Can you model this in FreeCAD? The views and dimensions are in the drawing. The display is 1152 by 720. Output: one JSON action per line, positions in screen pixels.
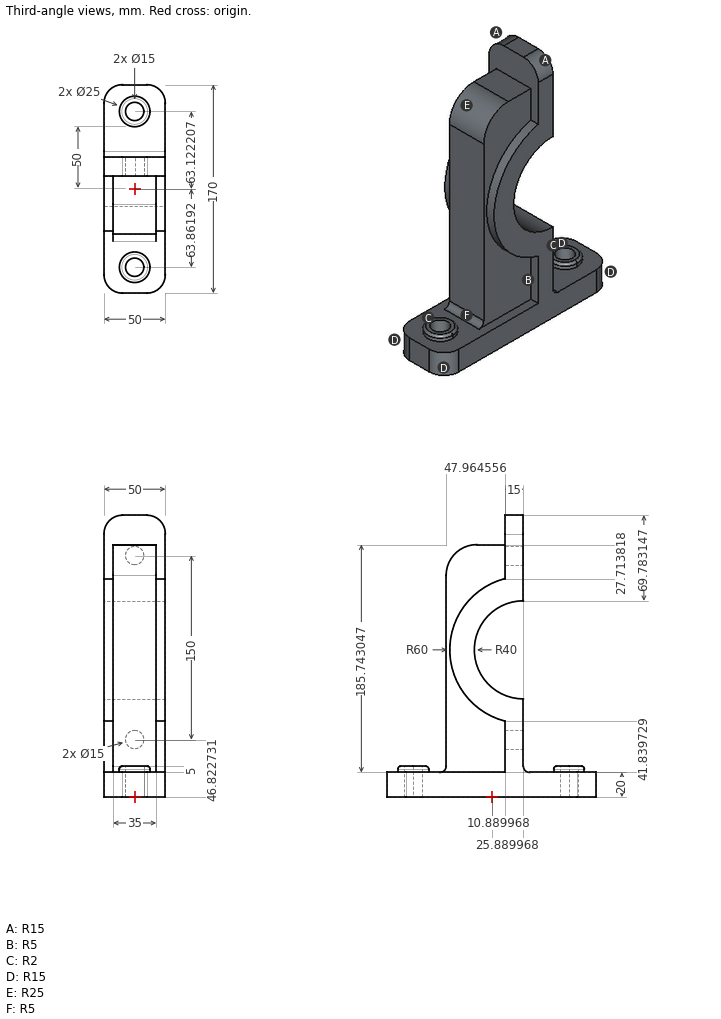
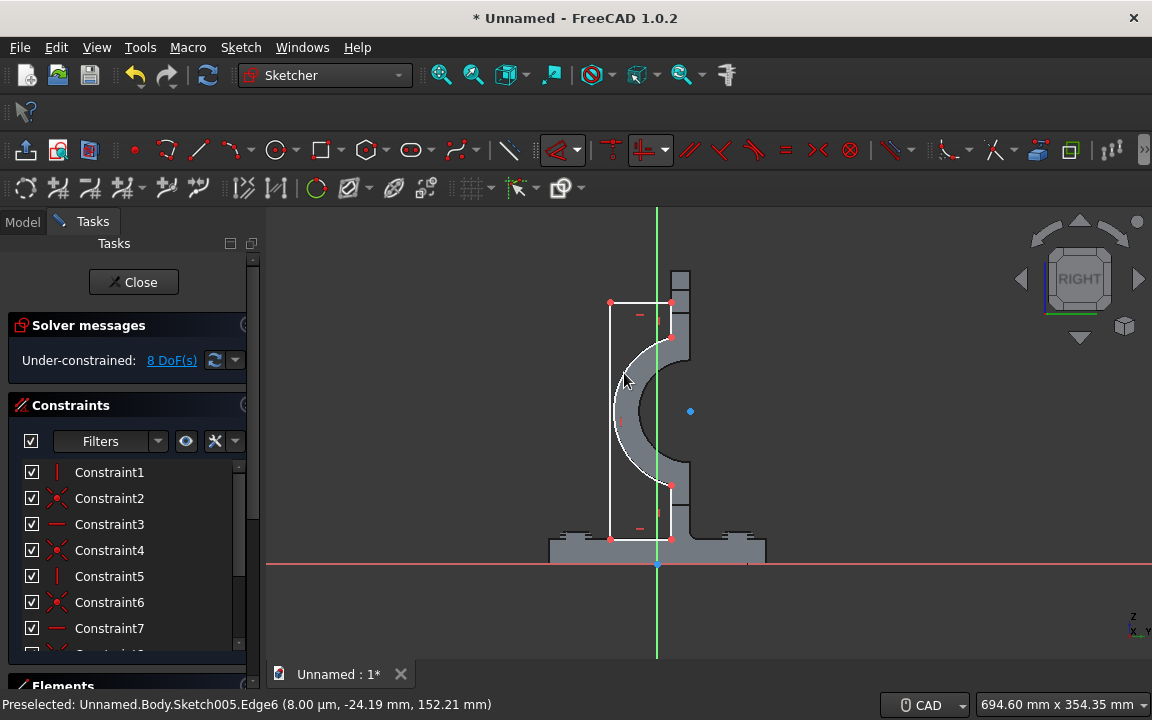
{"action": "left_click", "coordinate": [624, 374]}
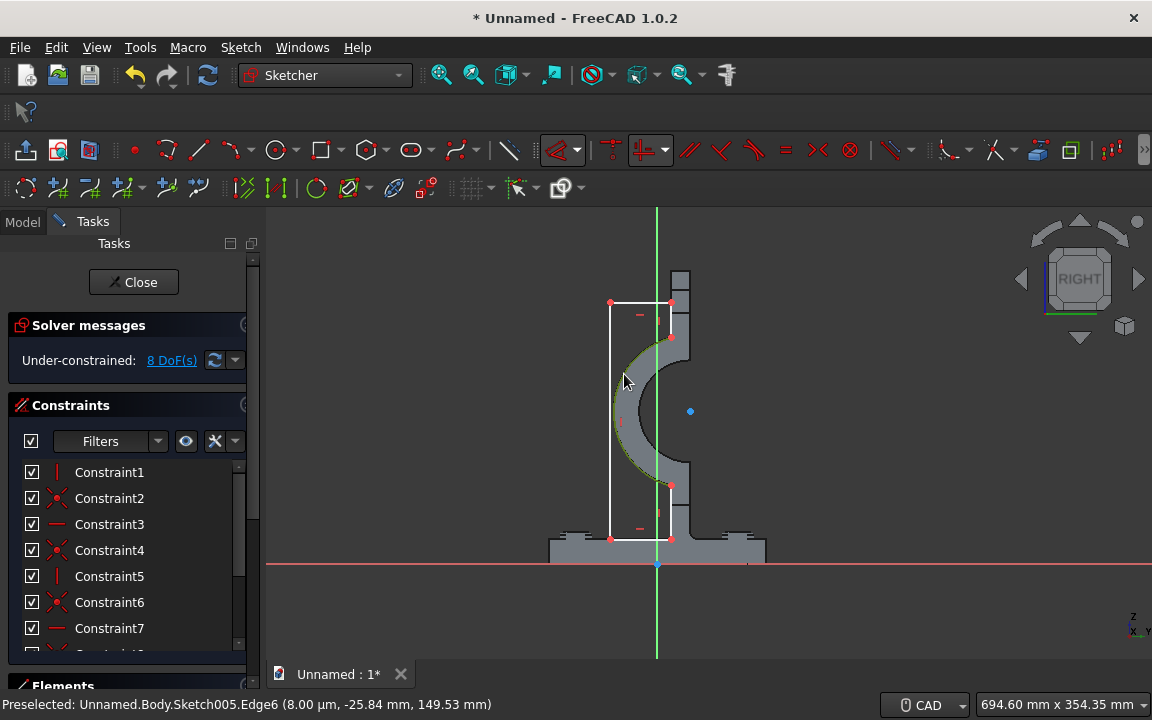
{"action": "key", "text": "k r"}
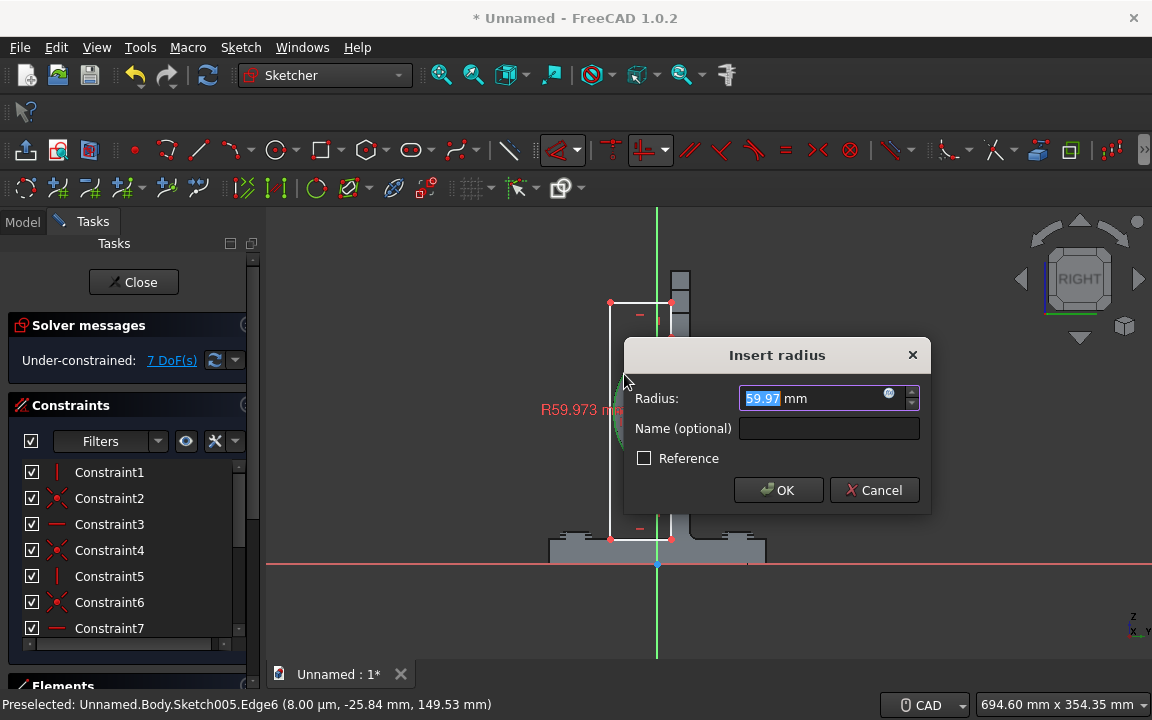
{"action": "type", "text": "60"}
{"action": "key", "text": "Return"}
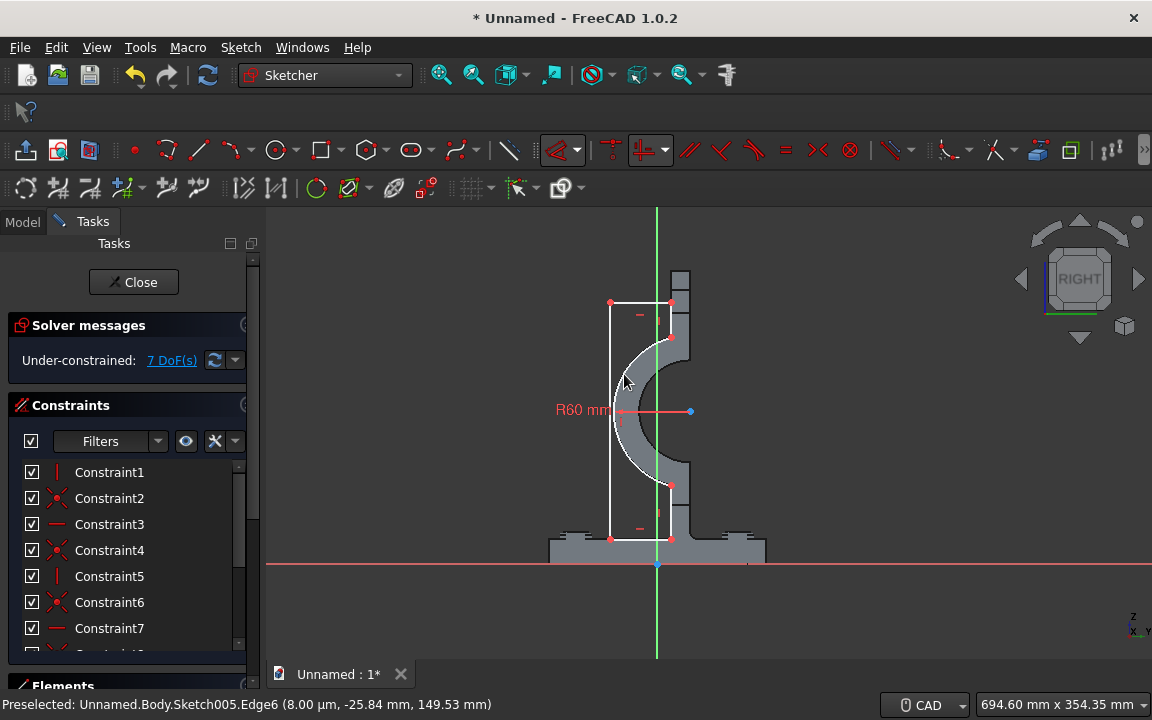
{"action": "scroll", "coordinate": [610, 540], "scroll_direction": "up", "scroll_amount": 3}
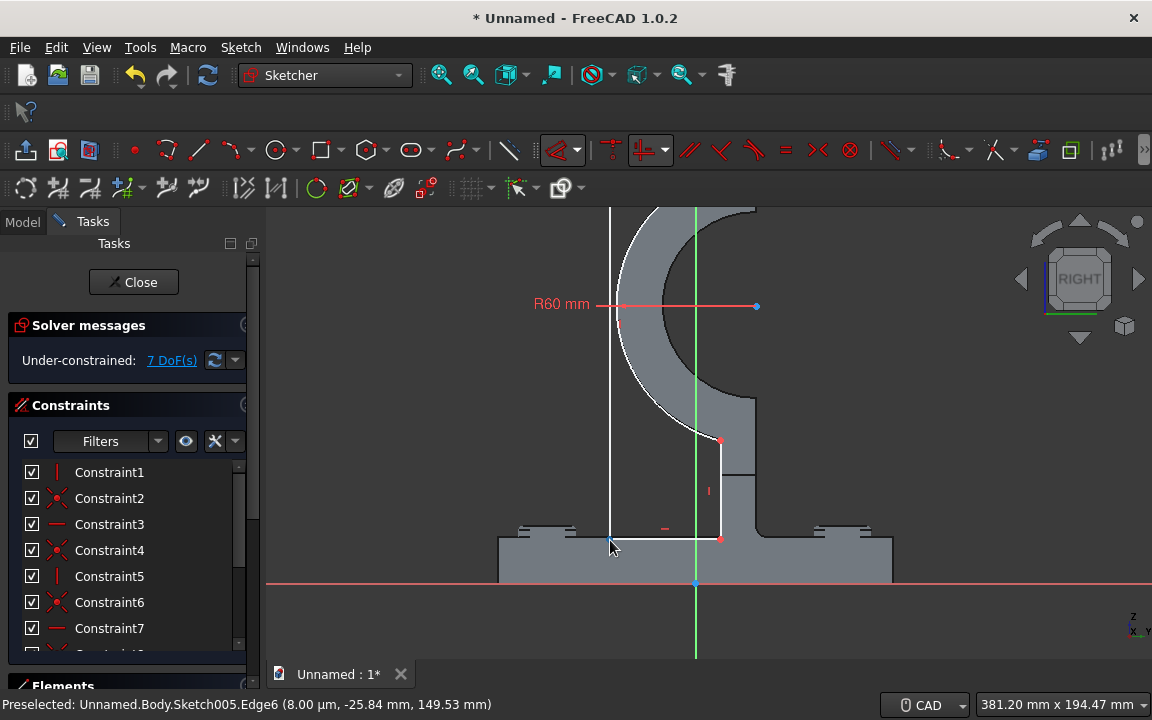
{"action": "left_click", "coordinate": [610, 539]}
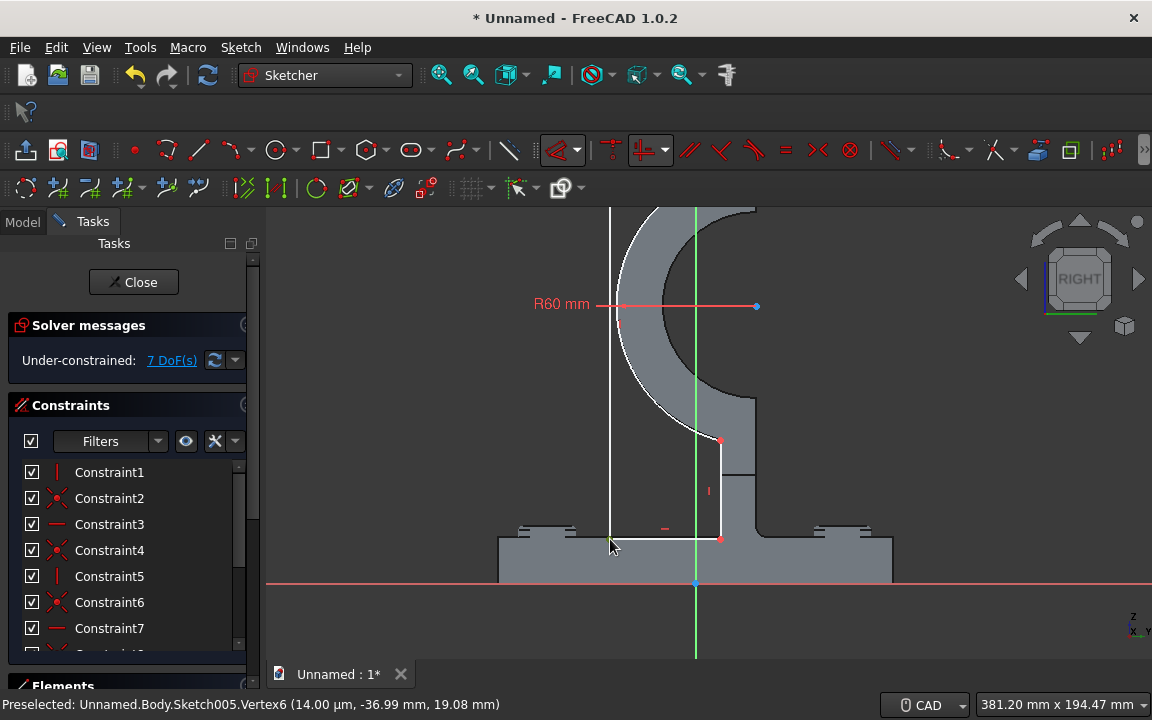
{"action": "left_click", "coordinate": [580, 150]}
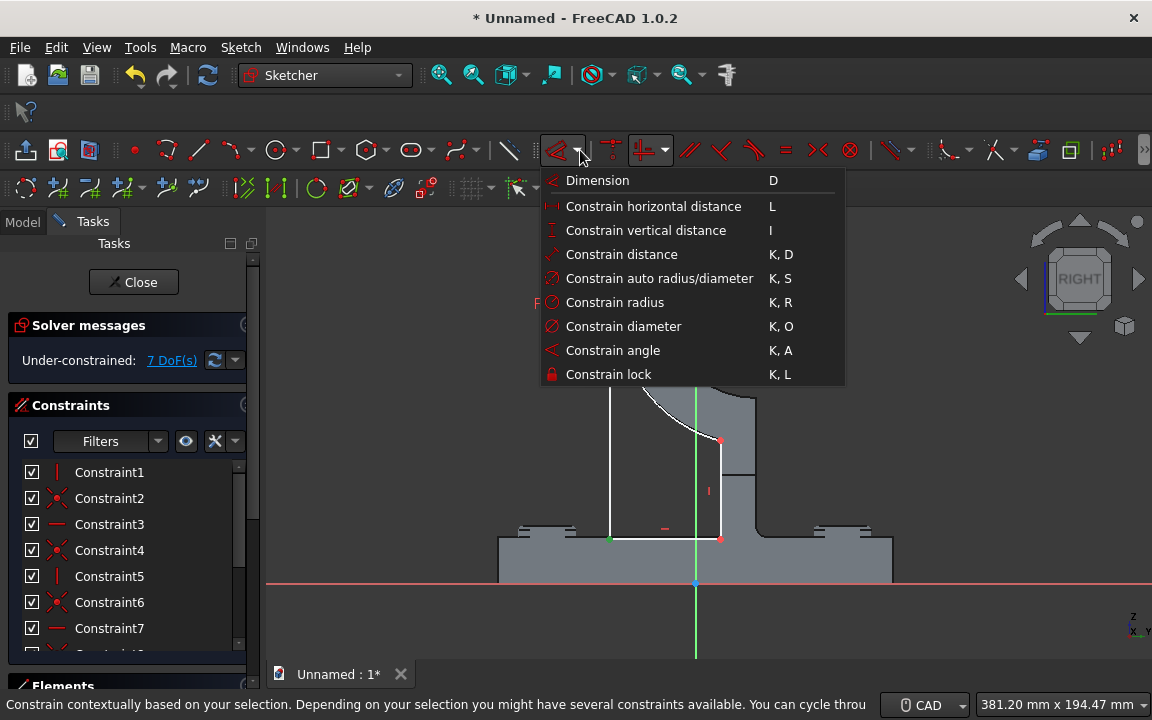
{"action": "left_click", "coordinate": [693, 230]}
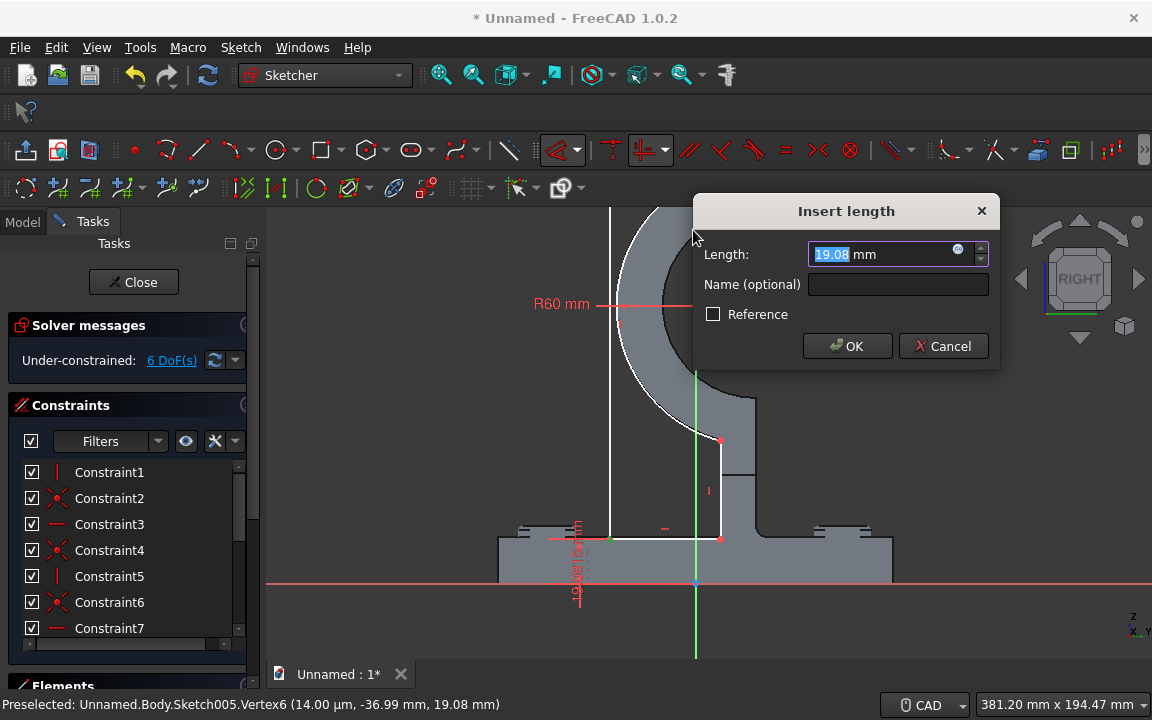
{"action": "type", "text": "20"}
{"action": "key", "text": "Return"}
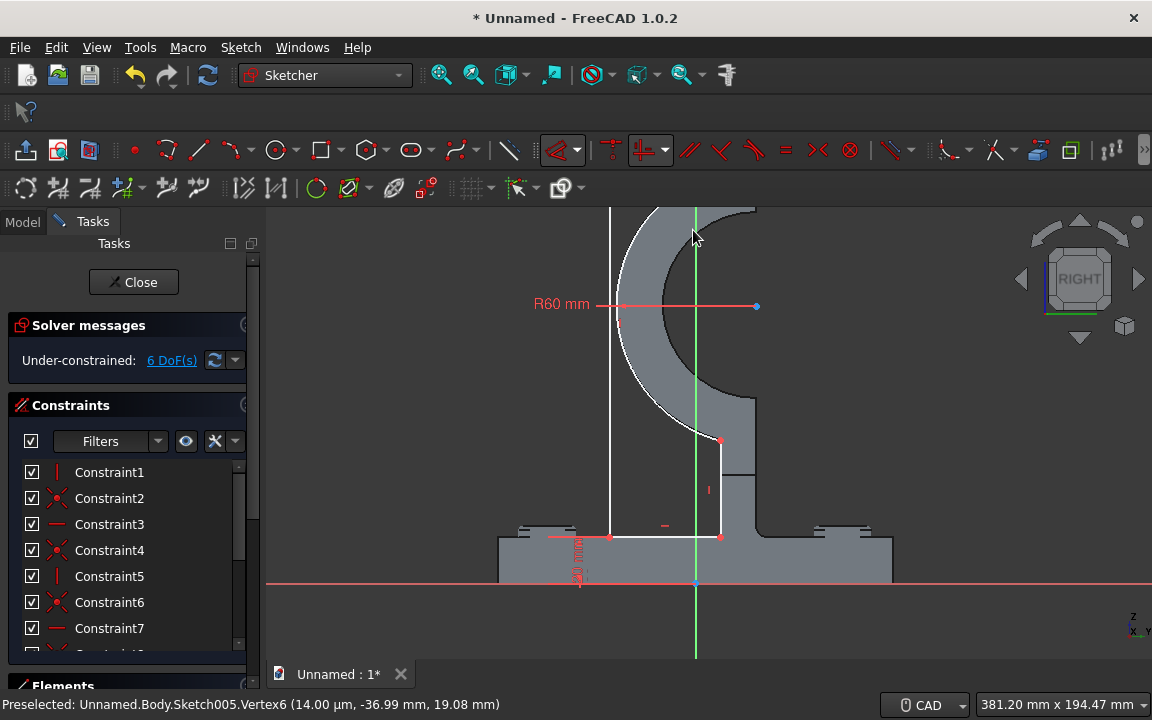
{"action": "scroll", "coordinate": [610, 540], "scroll_direction": "down", "scroll_amount": 3}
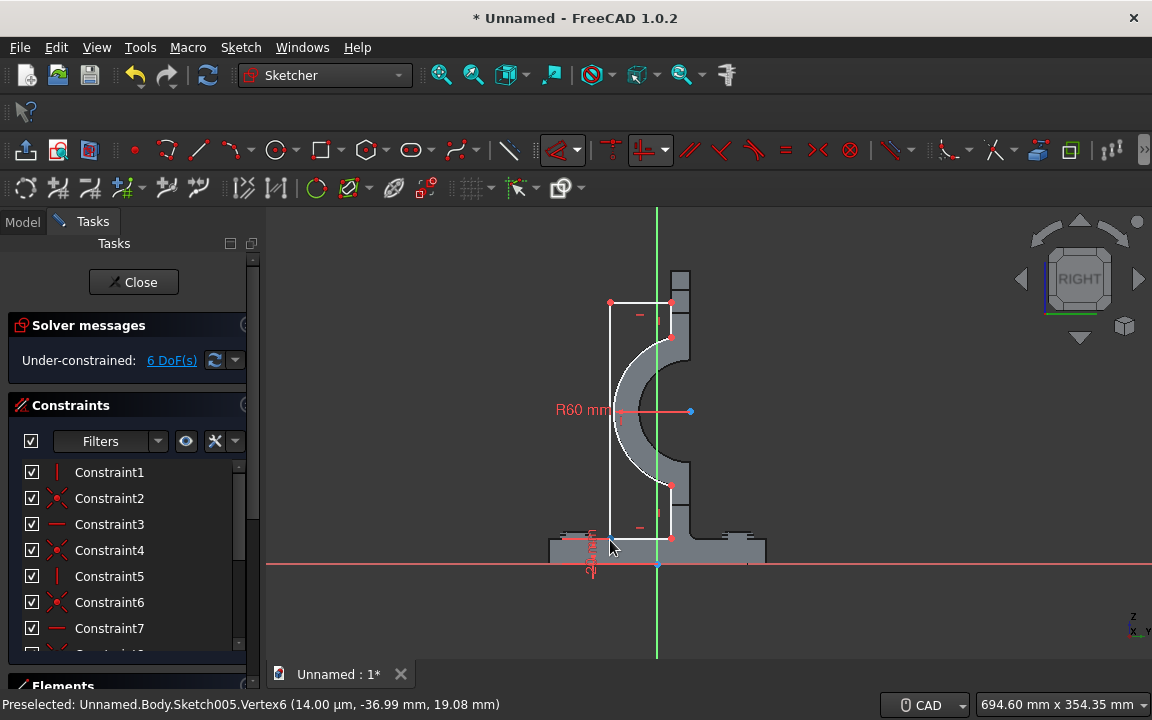
{"action": "scroll", "coordinate": [671, 327], "scroll_direction": "up", "scroll_amount": 2}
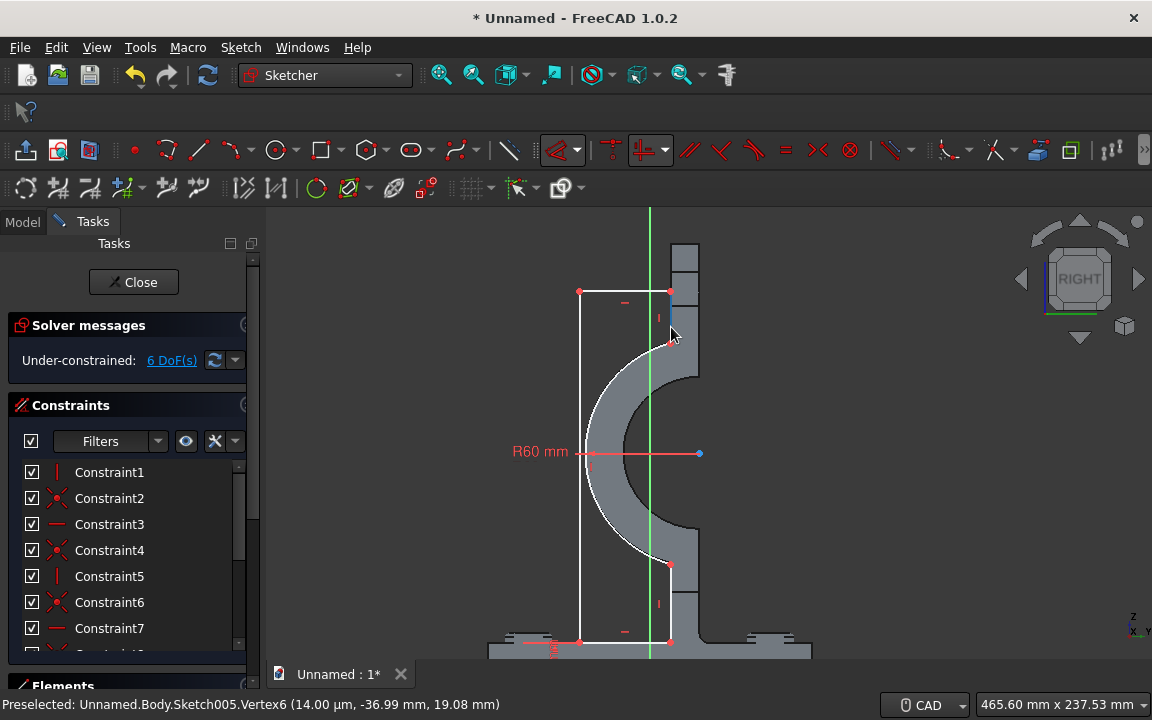
{"action": "left_click", "coordinate": [671, 328]}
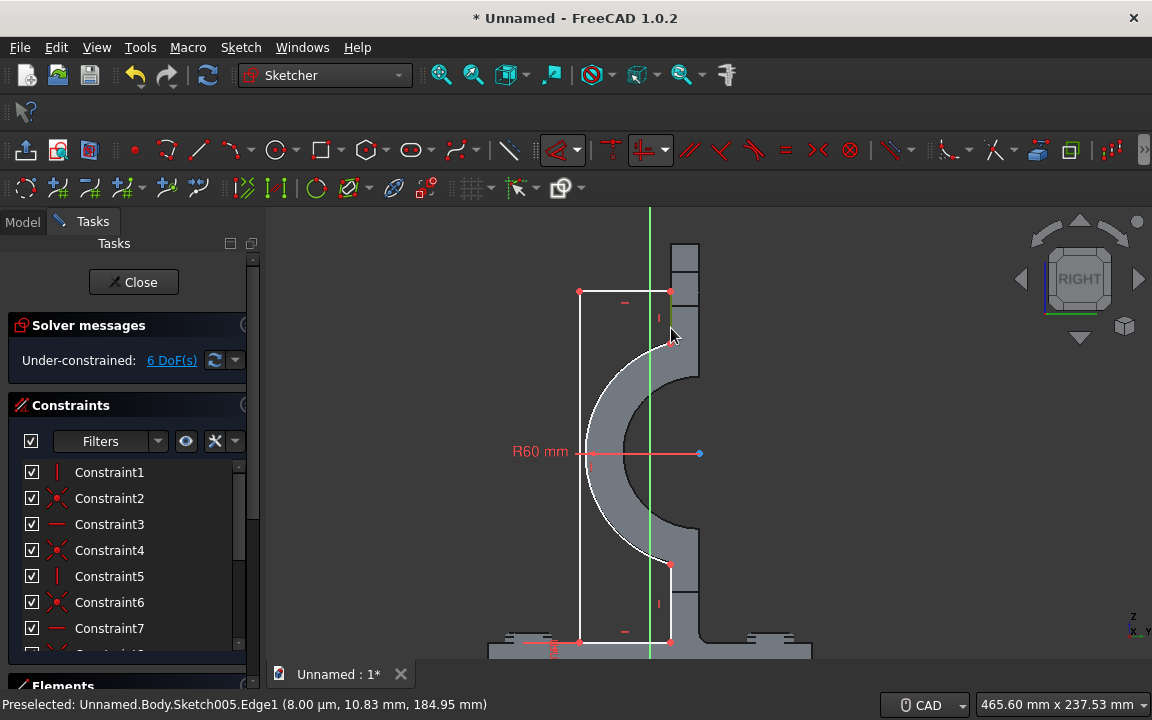
{"action": "key", "text": "i"}